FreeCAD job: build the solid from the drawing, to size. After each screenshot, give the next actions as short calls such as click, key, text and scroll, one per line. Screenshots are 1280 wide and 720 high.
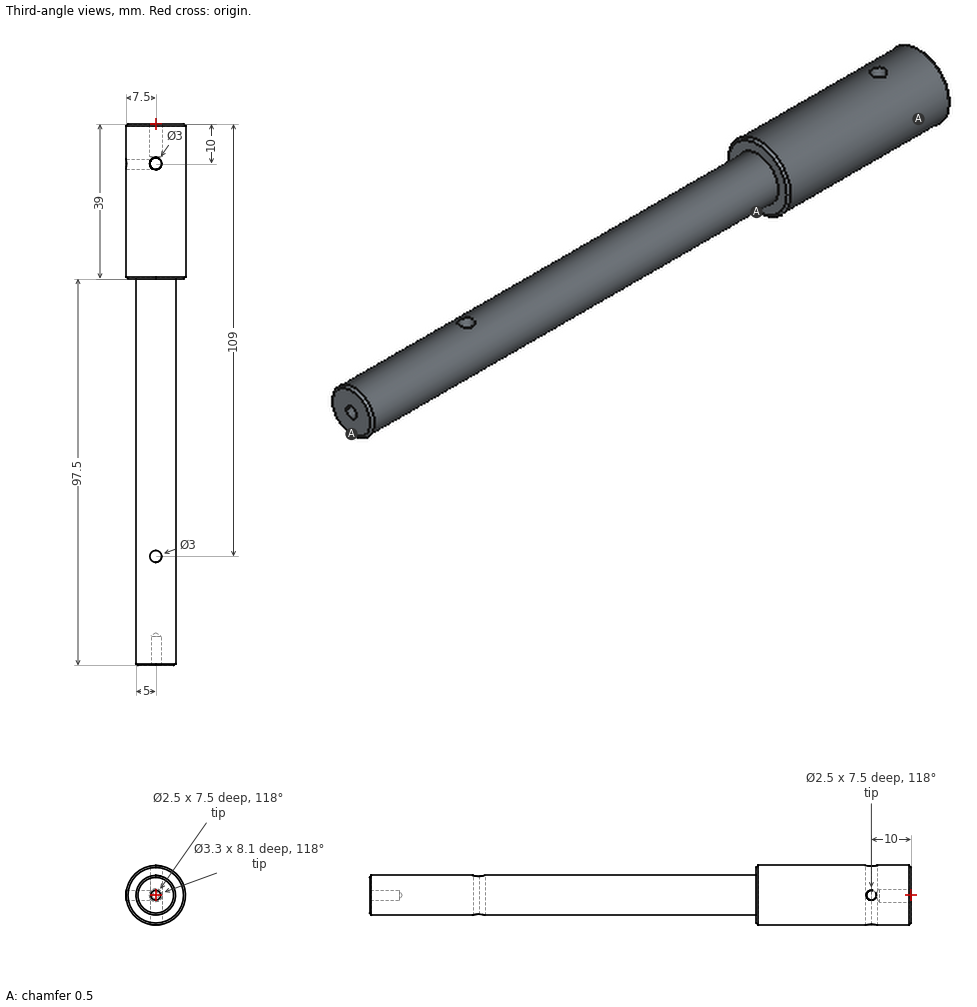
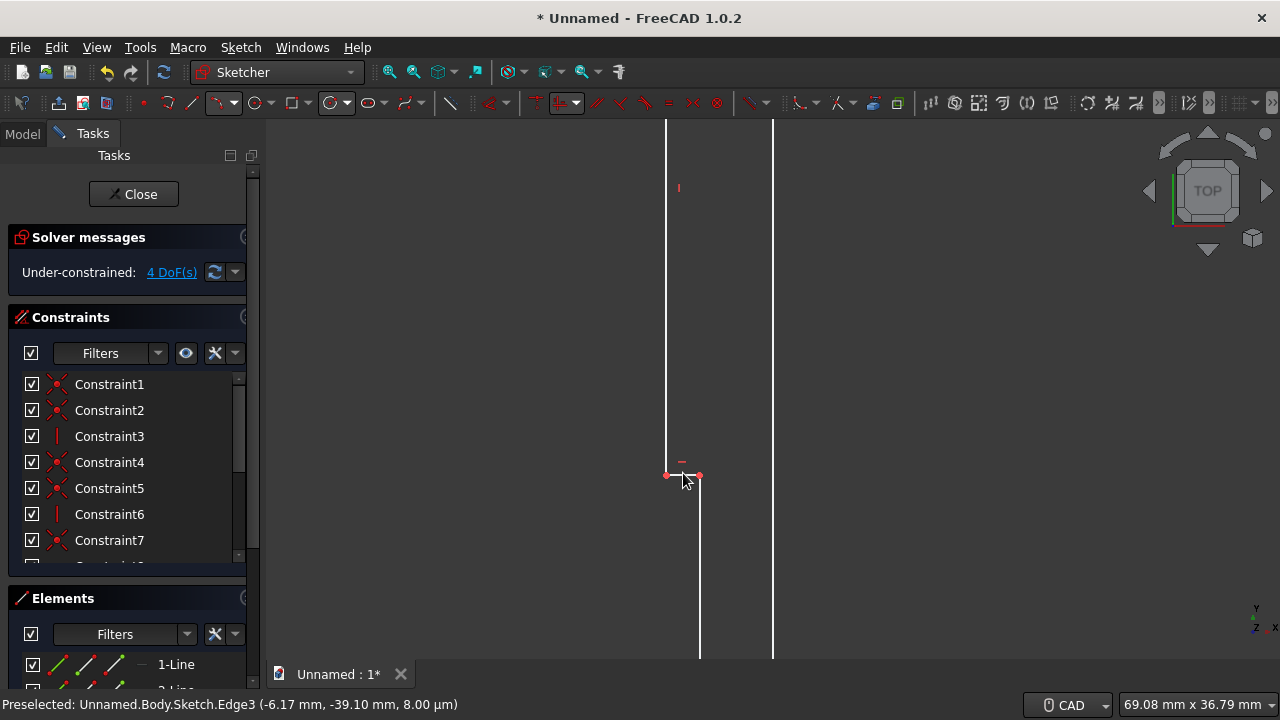
scroll(702, 288, down, 9)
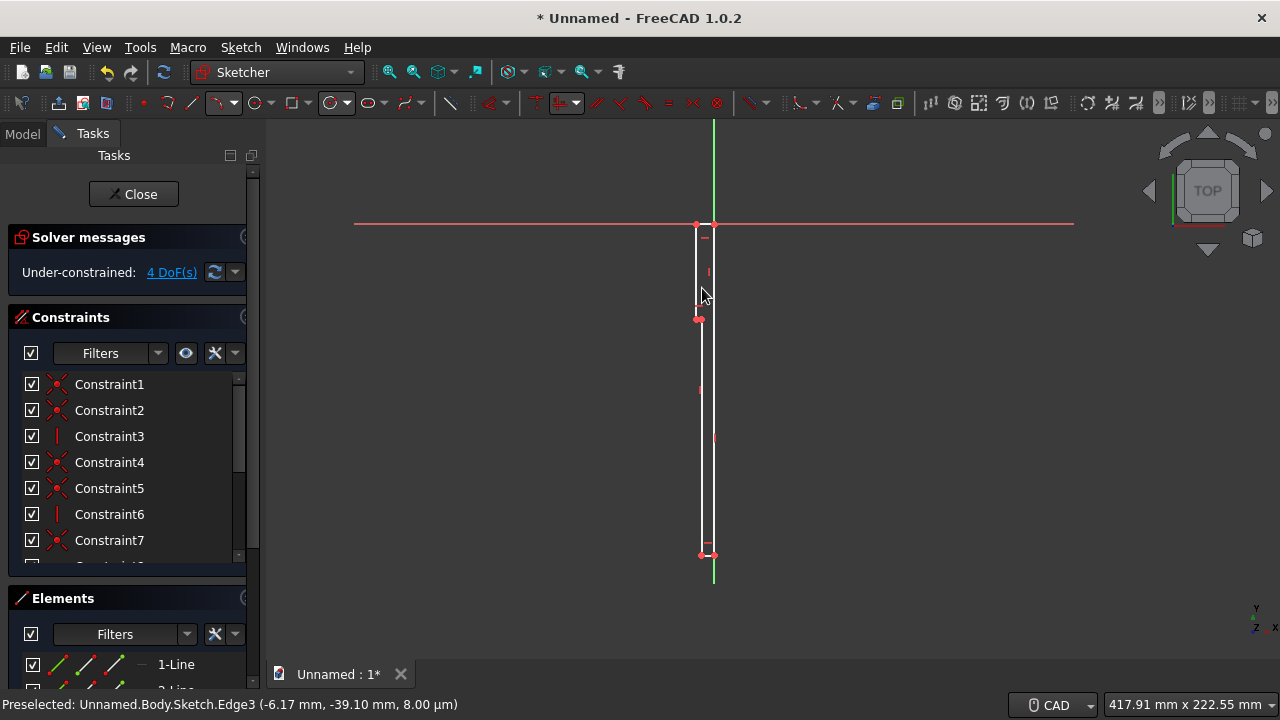
scroll(706, 556, up, 7)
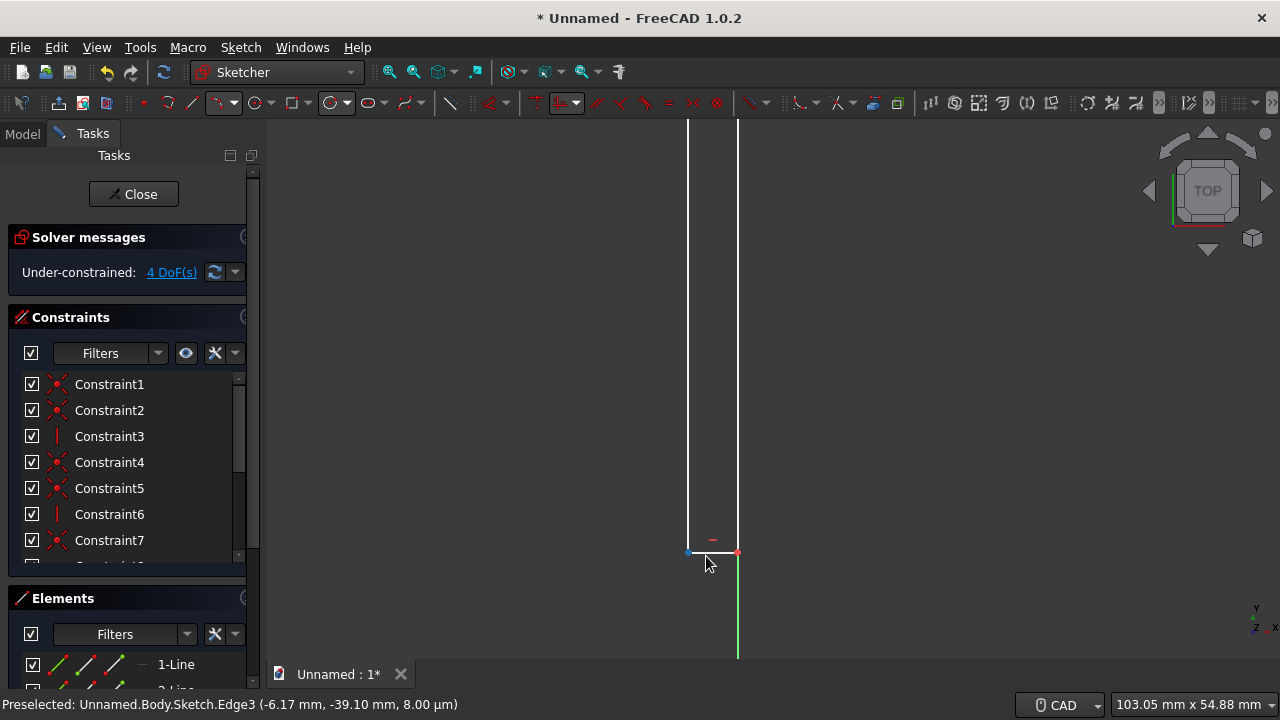
click(703, 553)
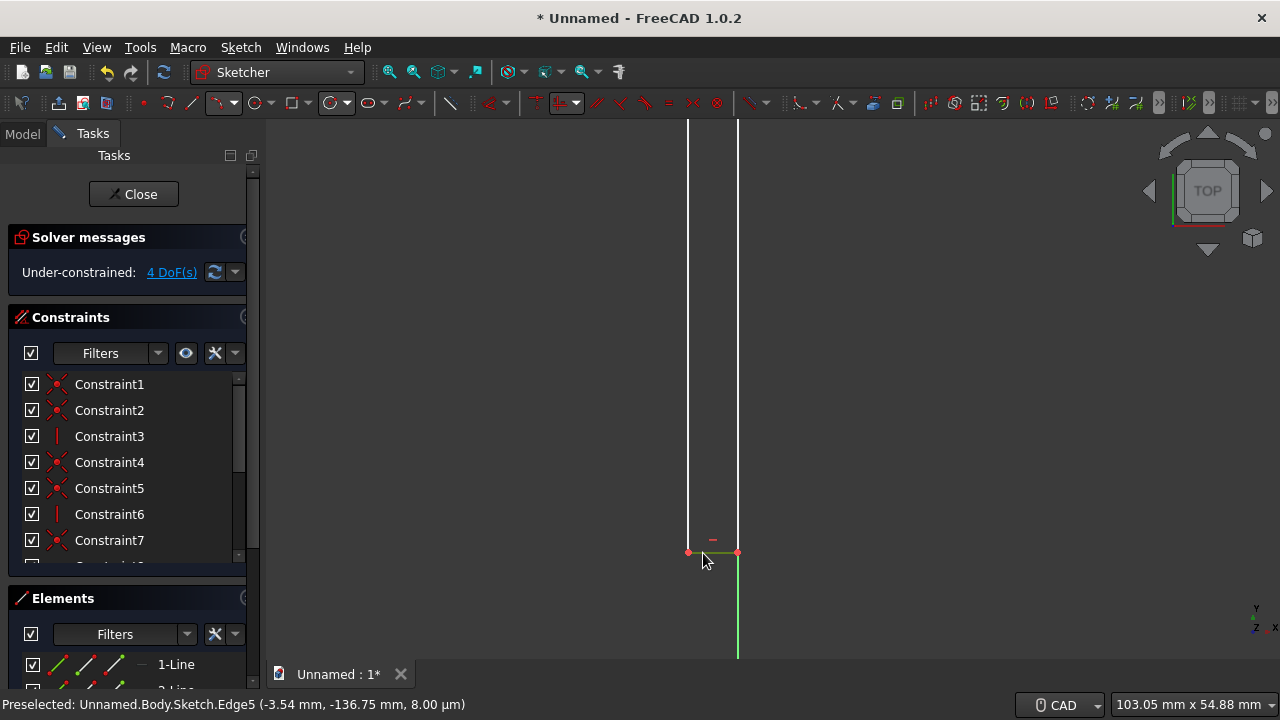
click(508, 104)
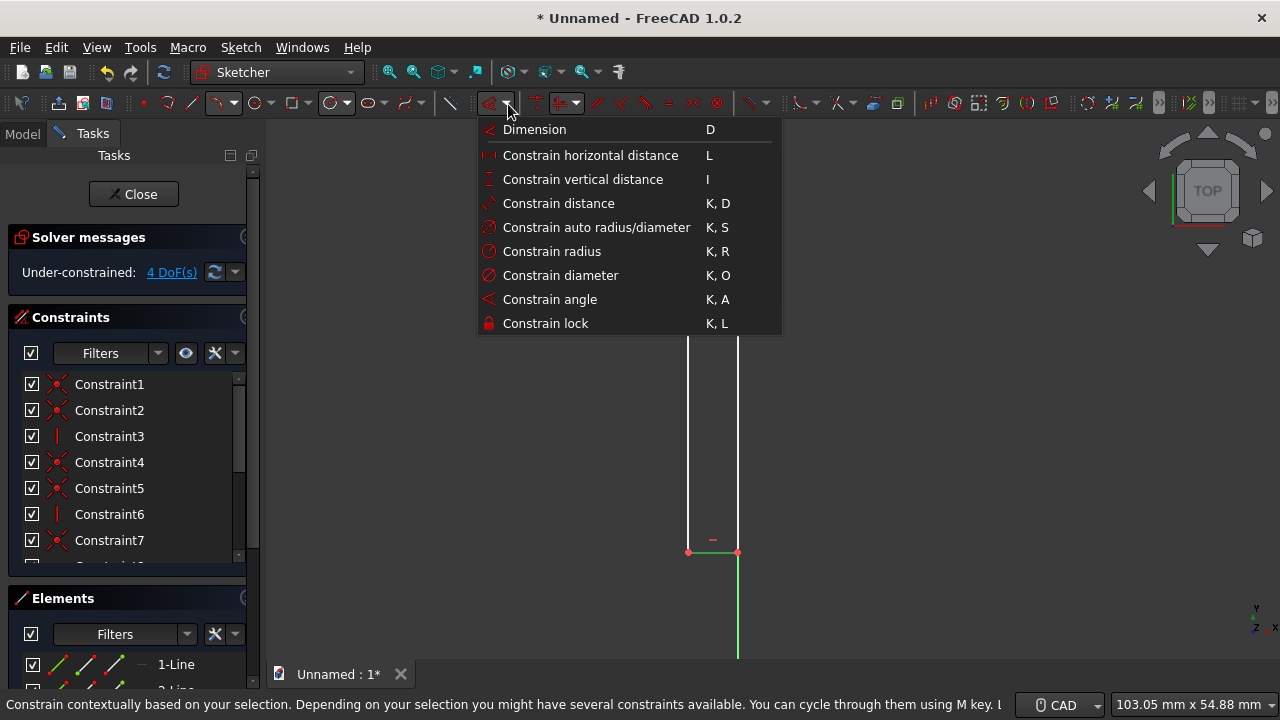
click(630, 155)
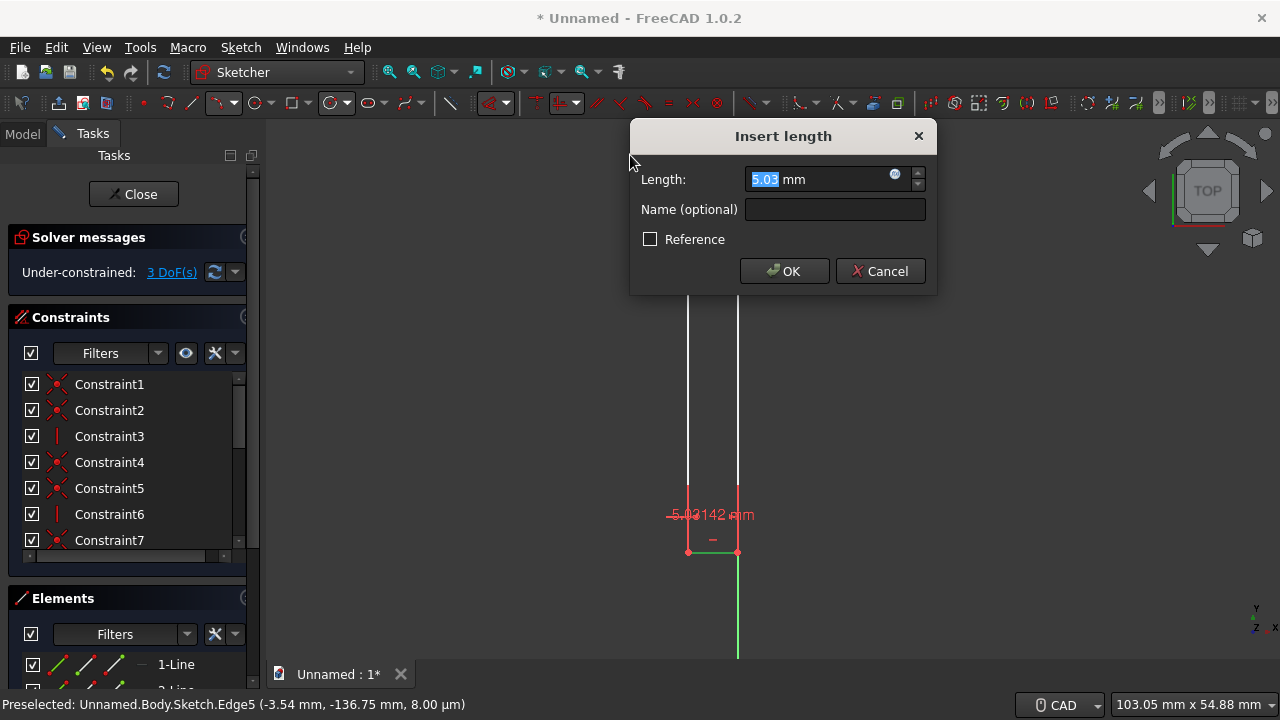
text(5)
key(Return)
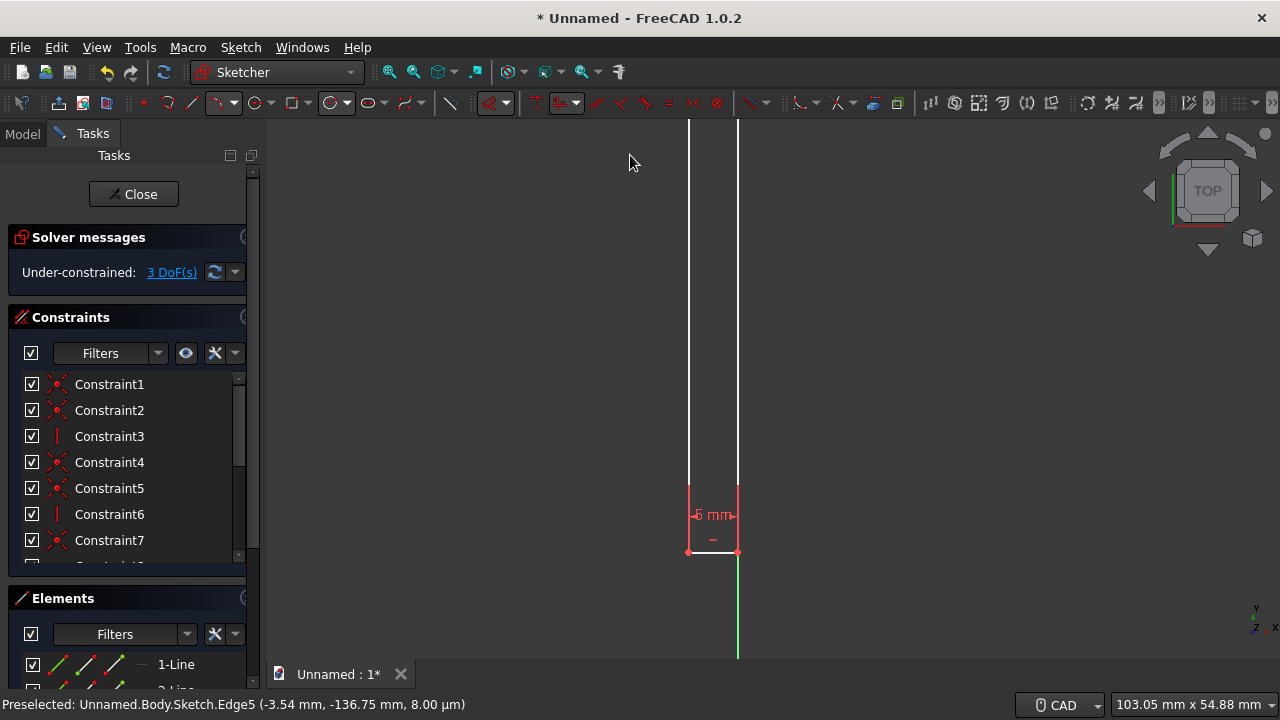
scroll(706, 556, down, 7)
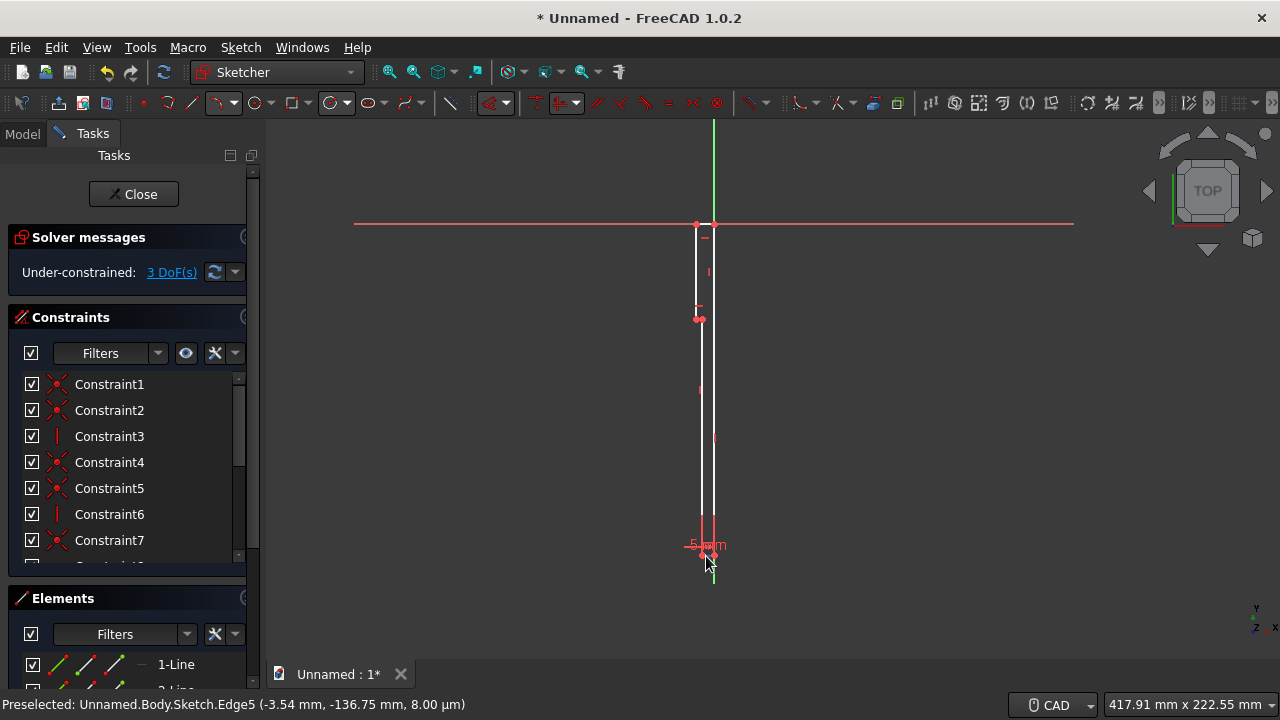
click(696, 253)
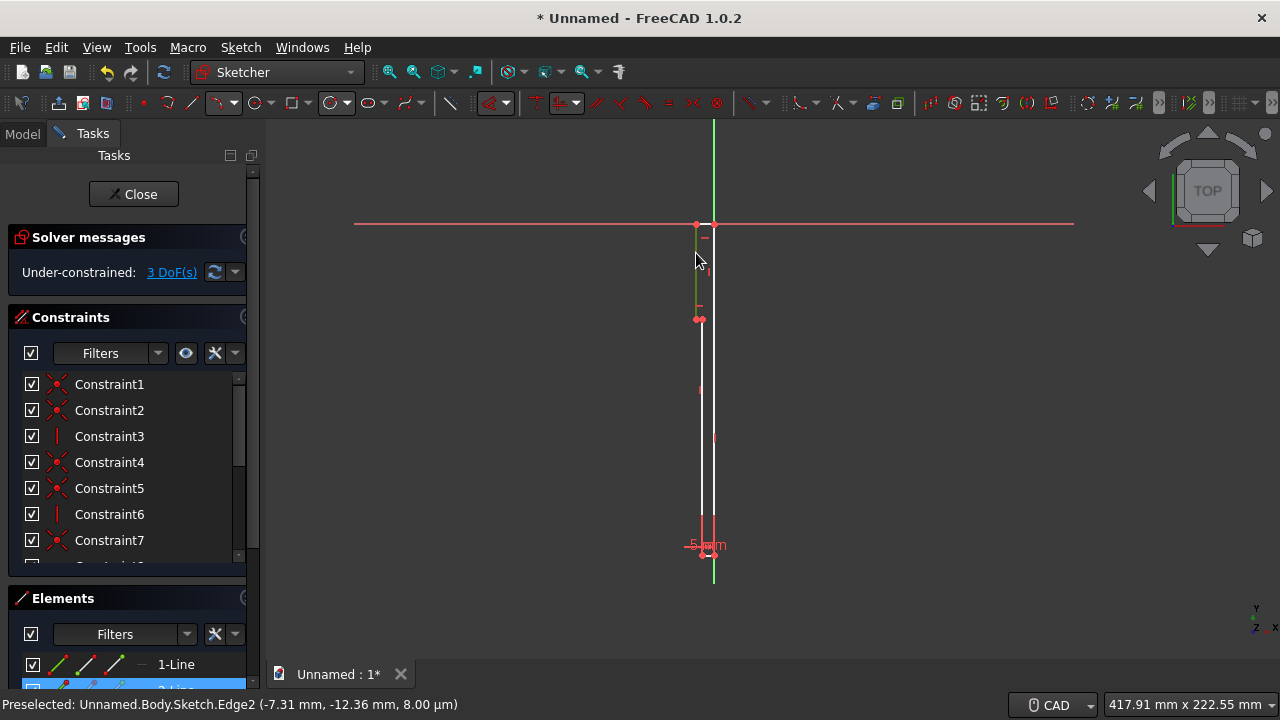
key(i)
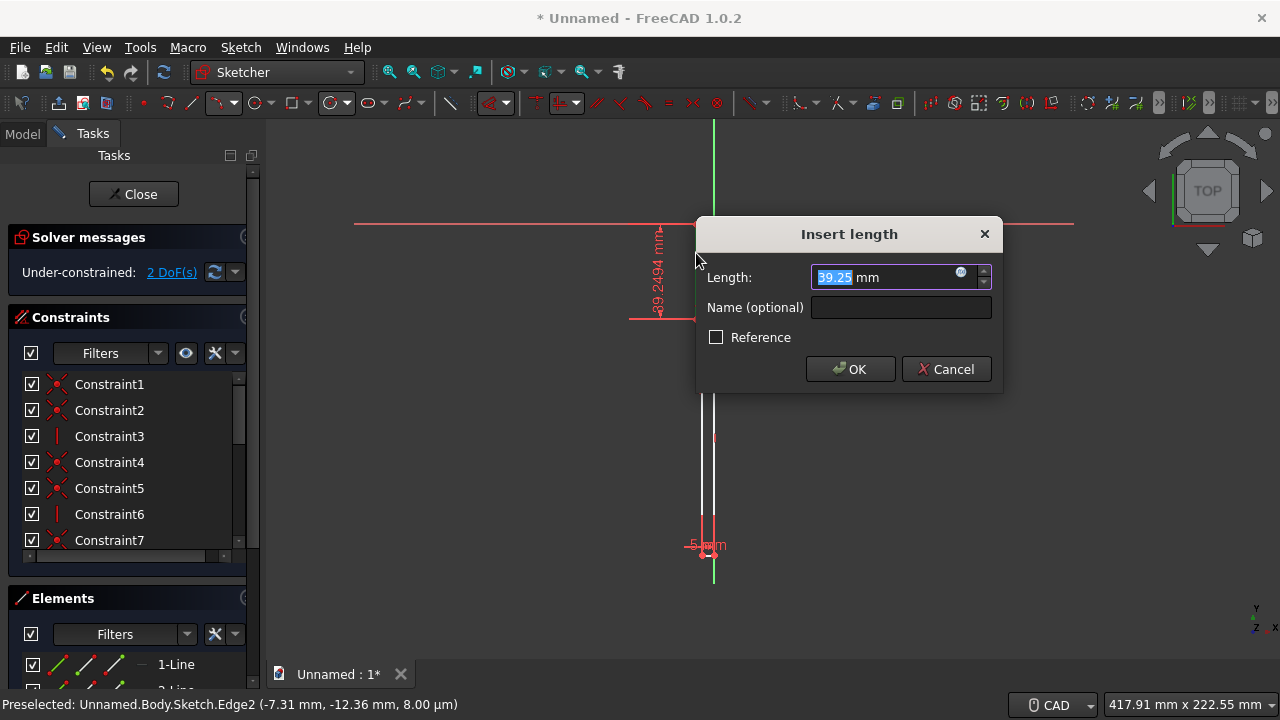
text(39)
key(Return)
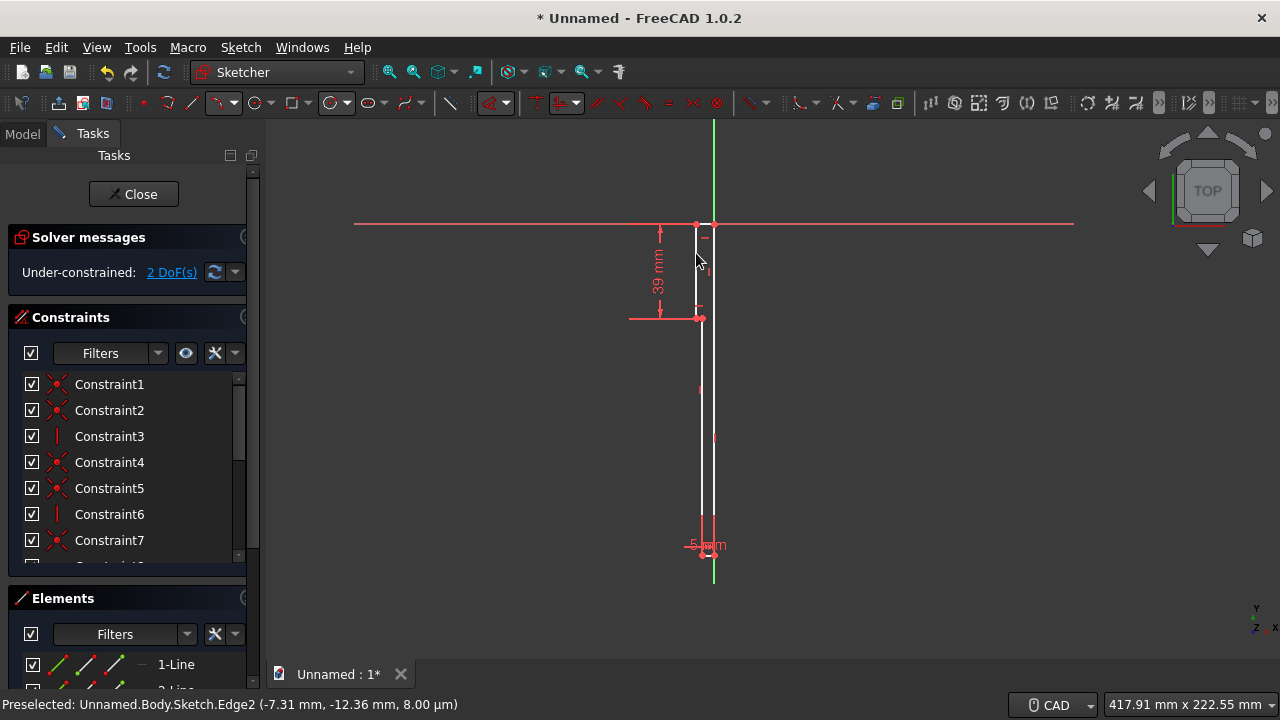
scroll(705, 224, up, 4)